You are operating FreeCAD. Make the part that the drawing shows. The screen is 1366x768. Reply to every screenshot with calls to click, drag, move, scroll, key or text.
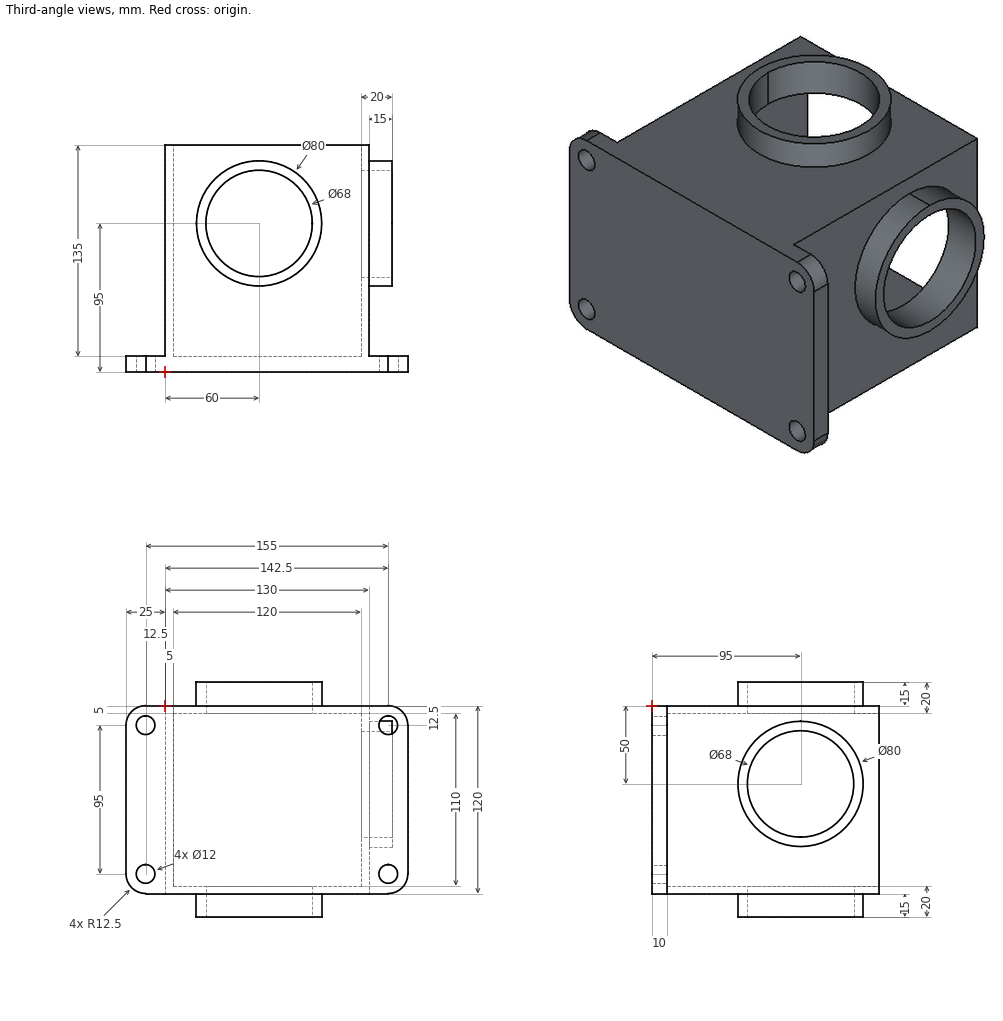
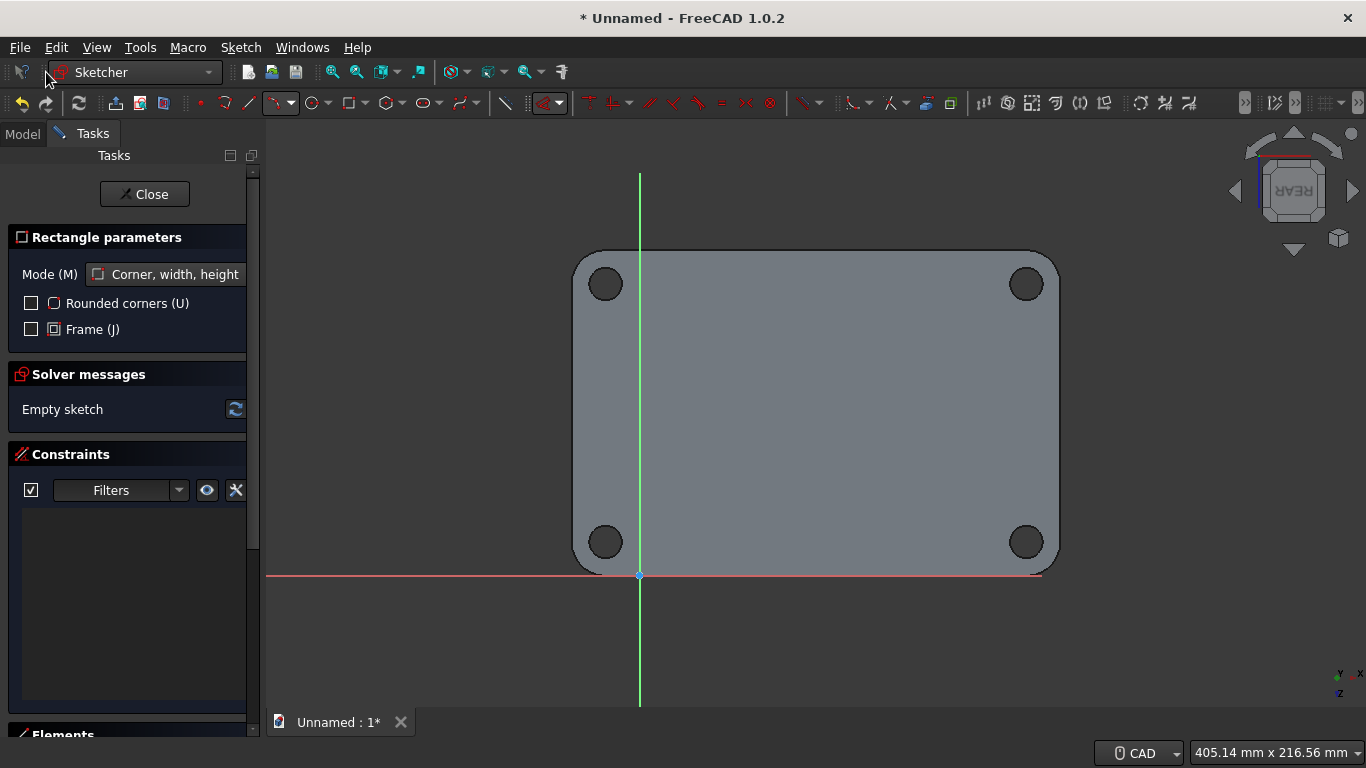
click(640, 576)
move(992, 250)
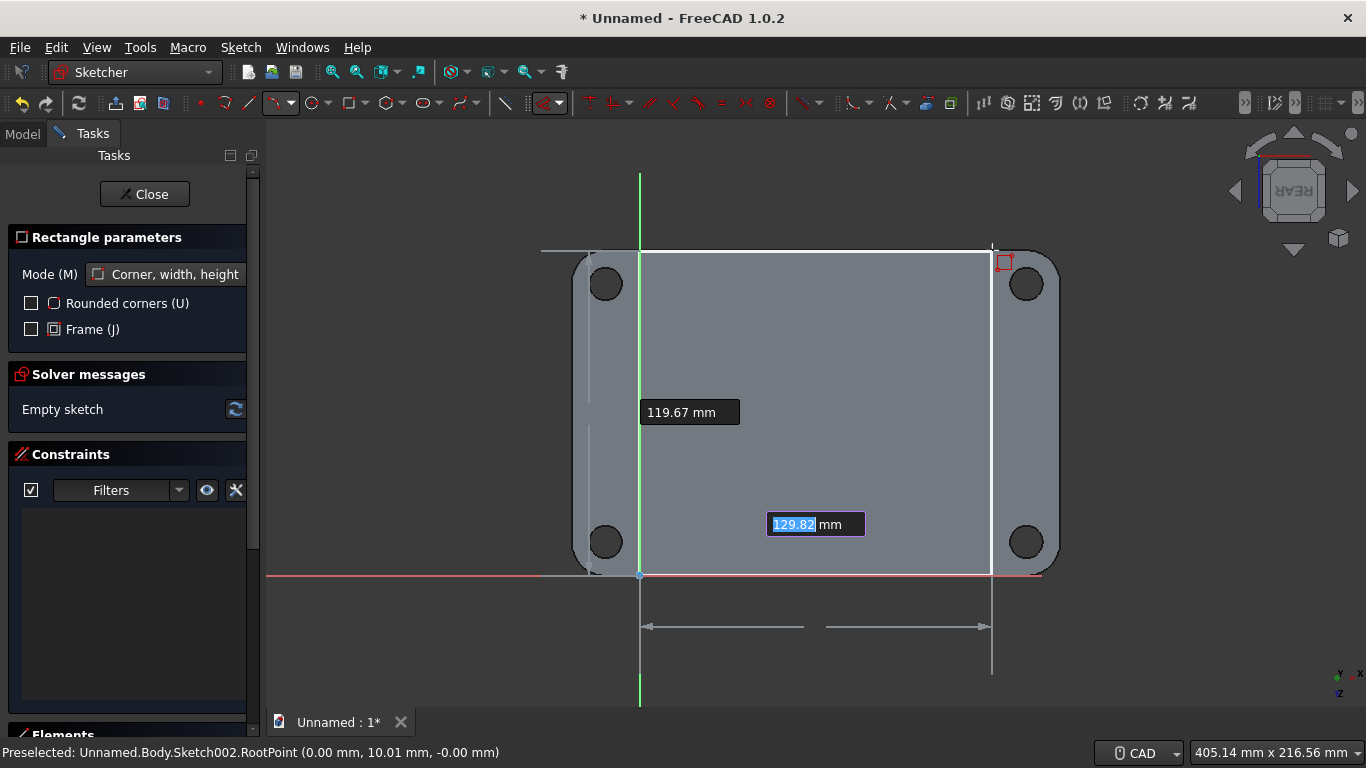
text(130)
key(Tab)
text(120)
key(Return)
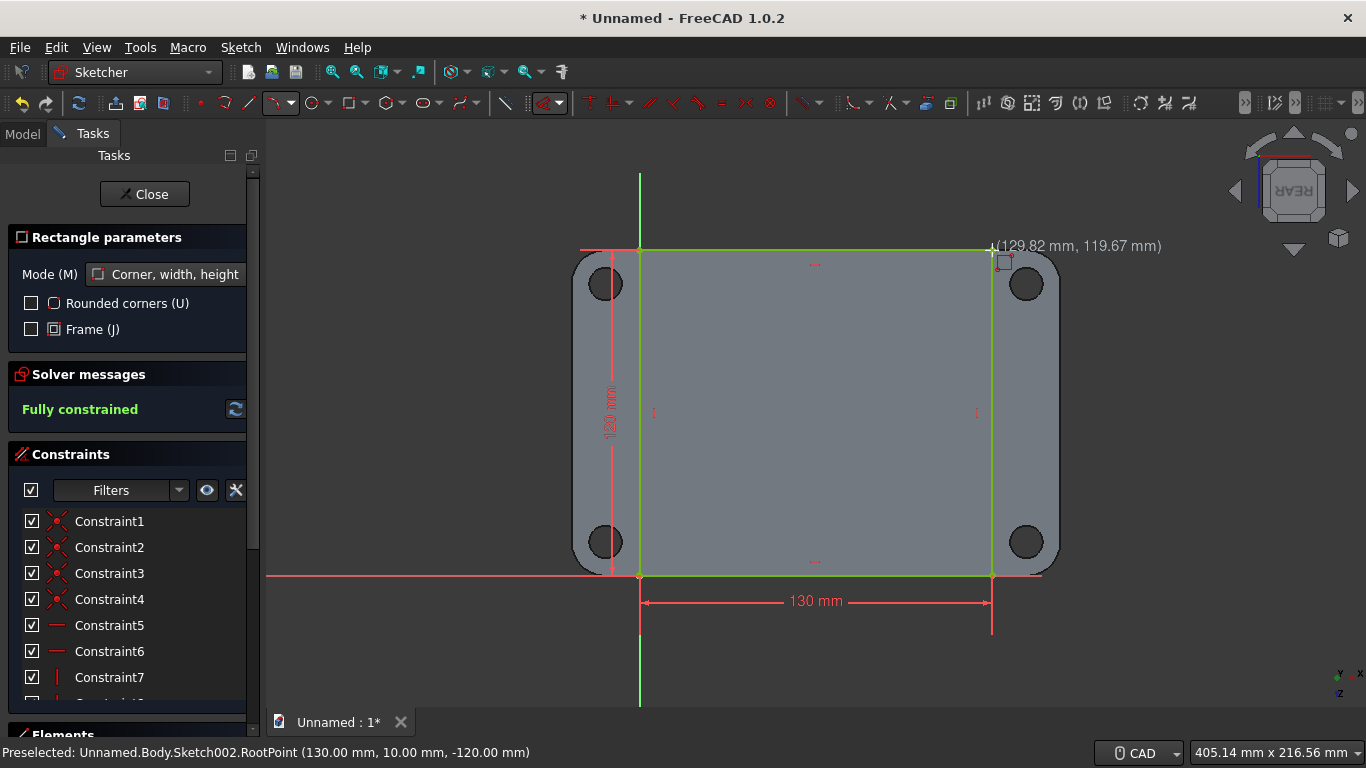
click(653, 264)
move(979, 562)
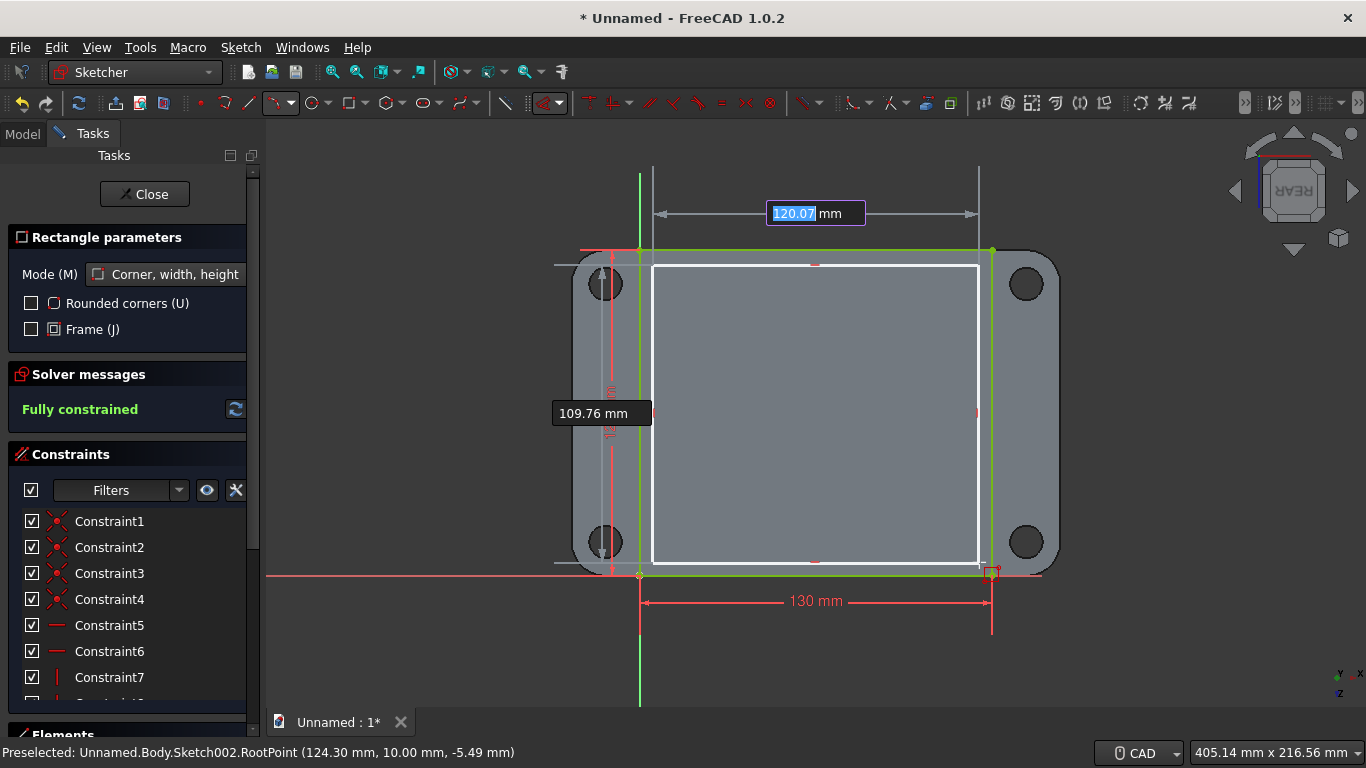
text(120)
key(Tab)
text(110)
key(Return)
key(Escape)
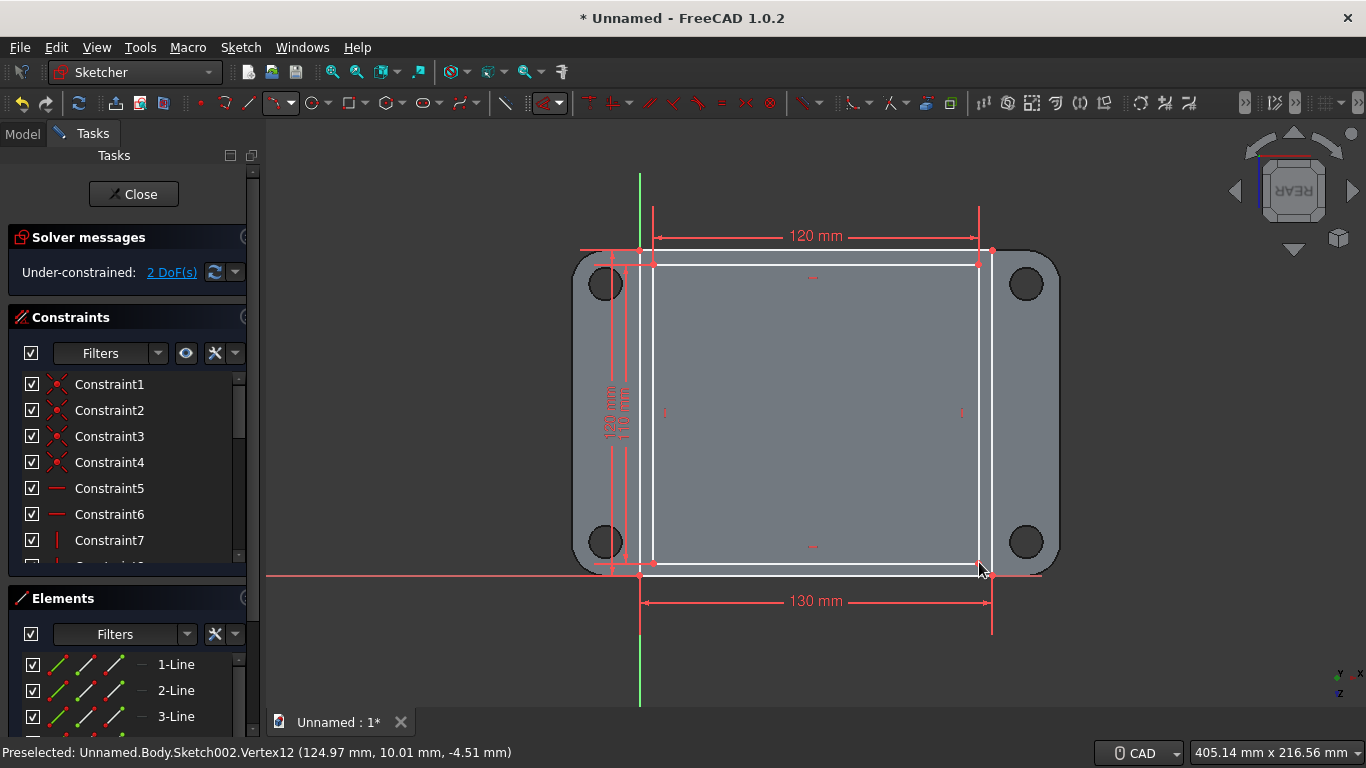
scroll(653, 265, up, 6)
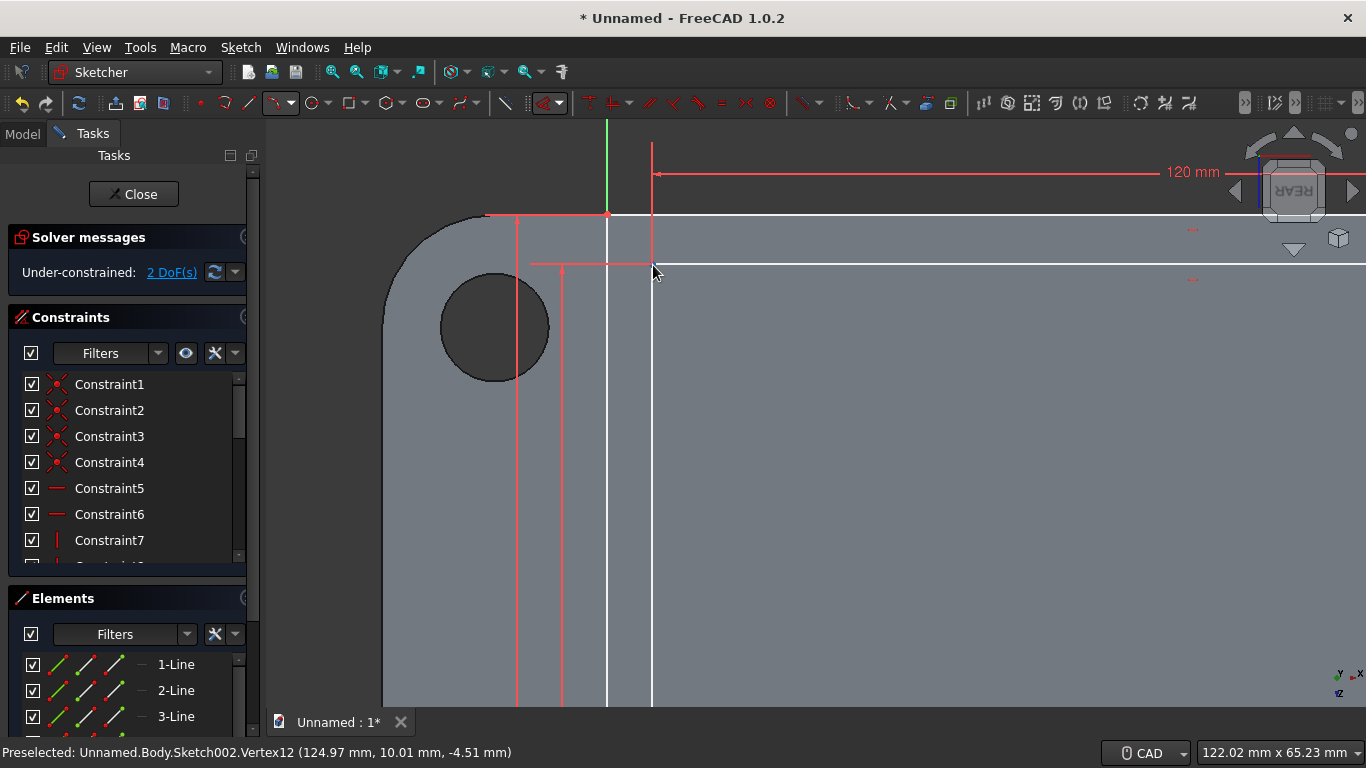
click(652, 264)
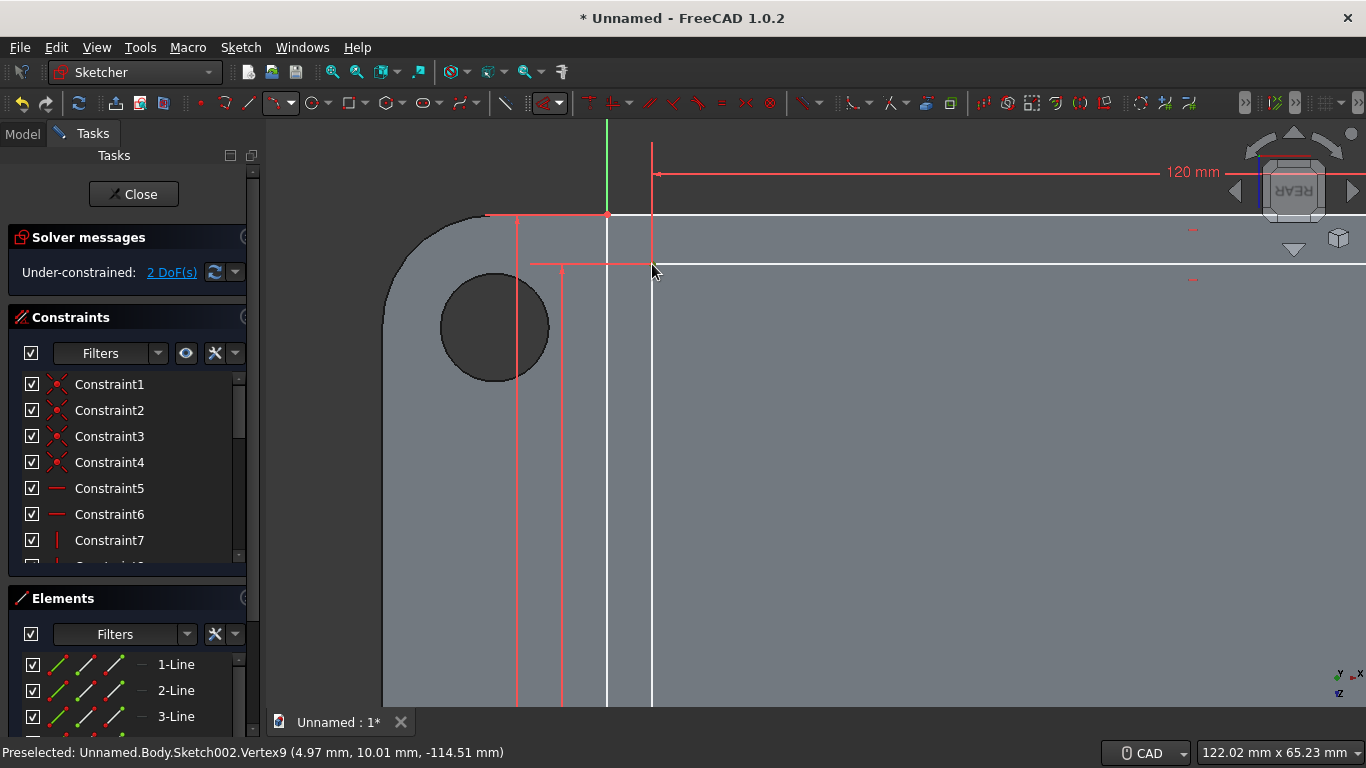
click(562, 104)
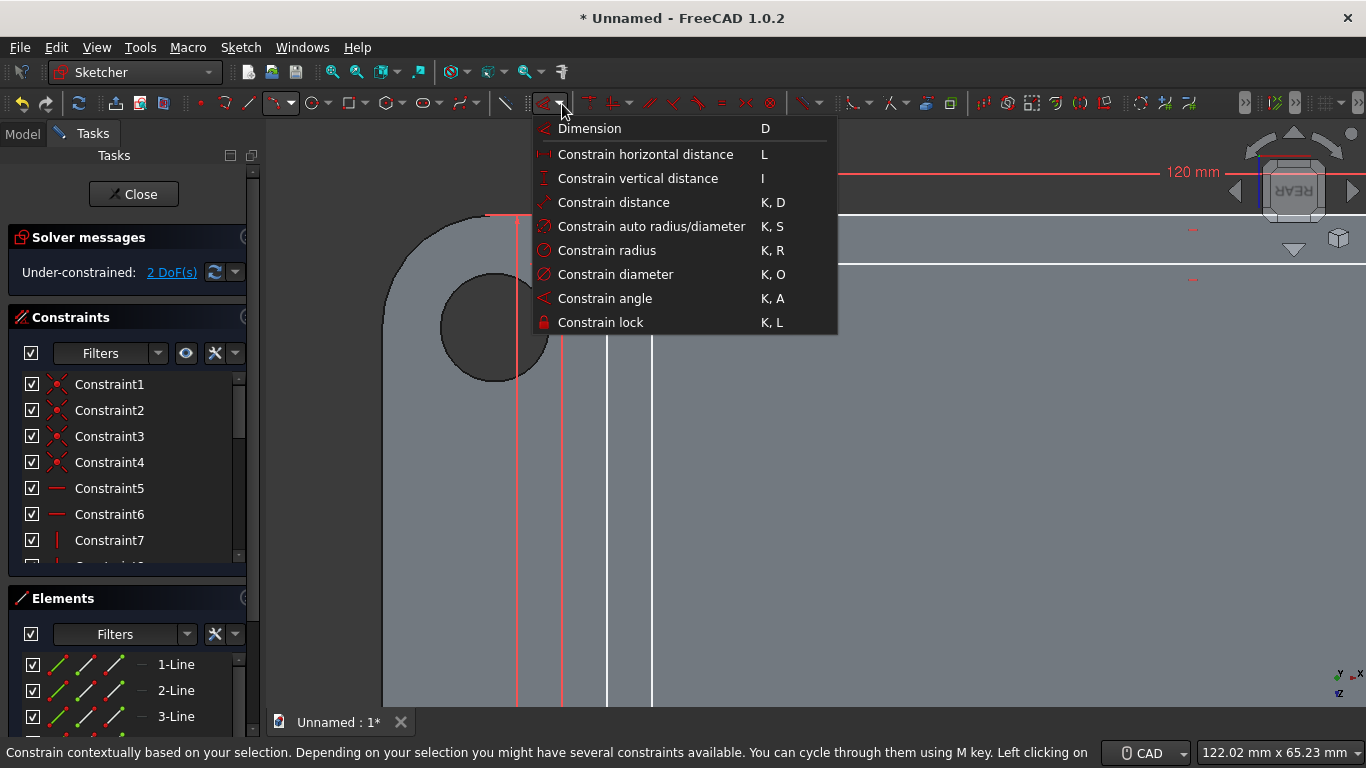
click(685, 154)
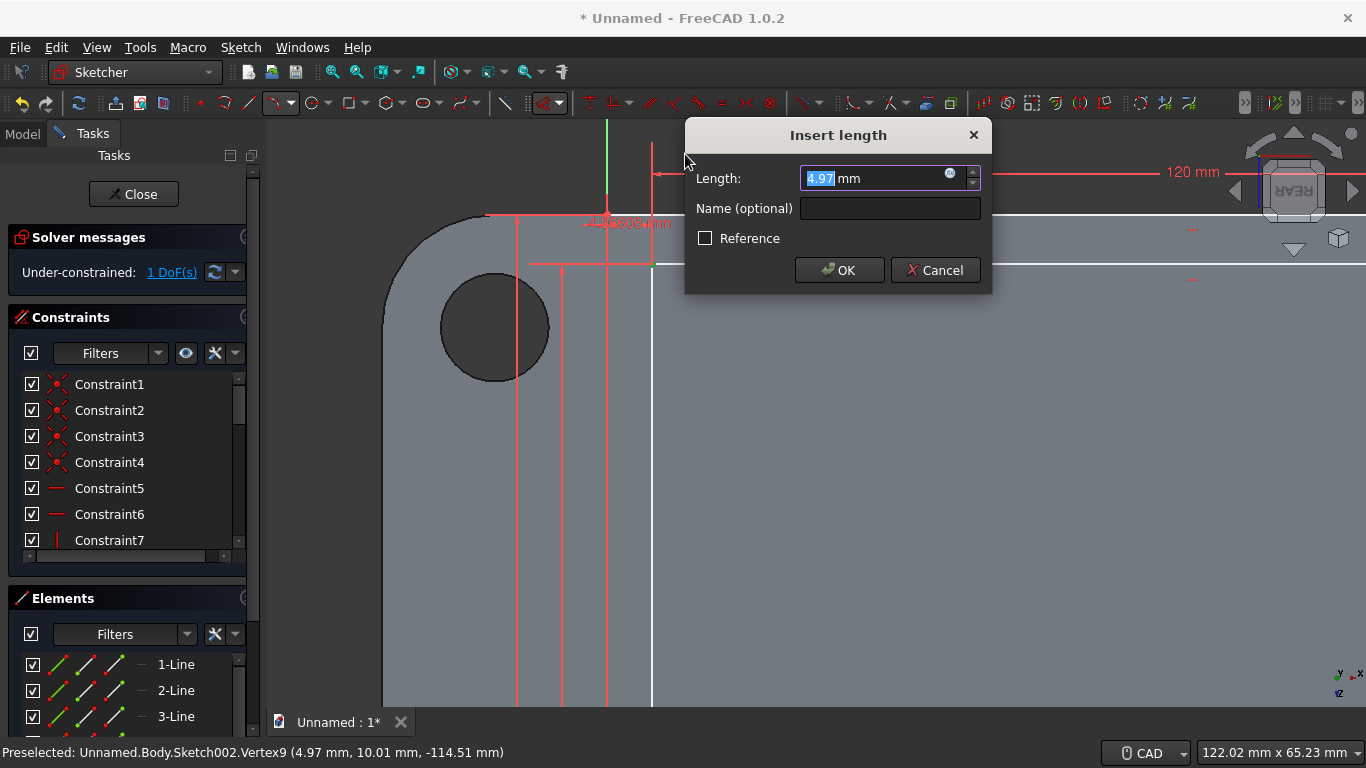
text(5)
key(Return)